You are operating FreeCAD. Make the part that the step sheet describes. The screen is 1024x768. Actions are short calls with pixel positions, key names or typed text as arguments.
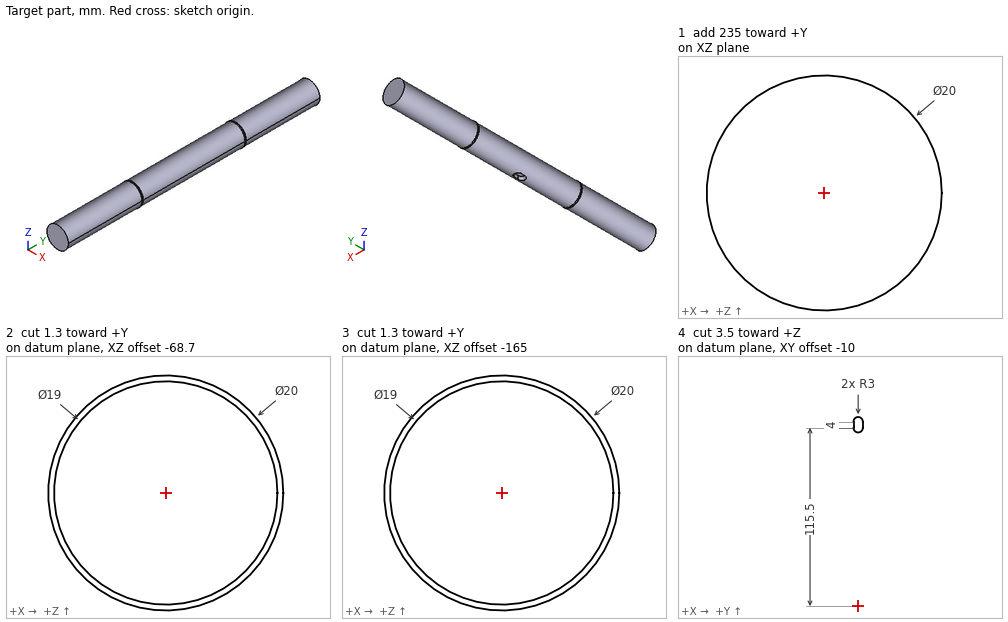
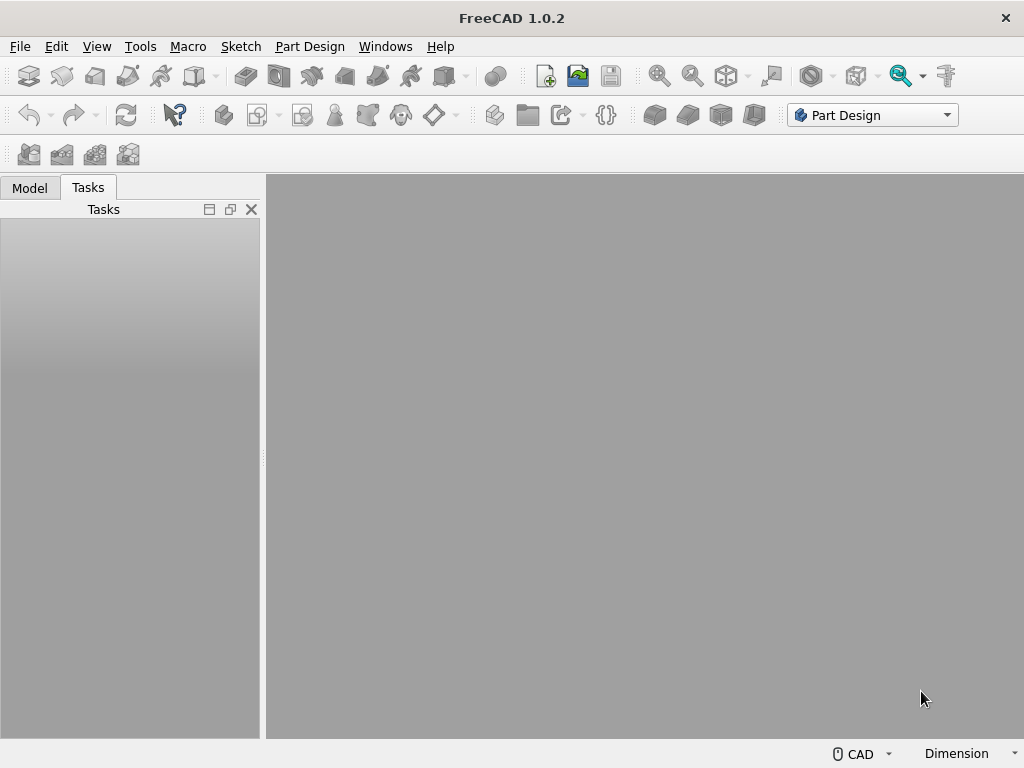
click(545, 76)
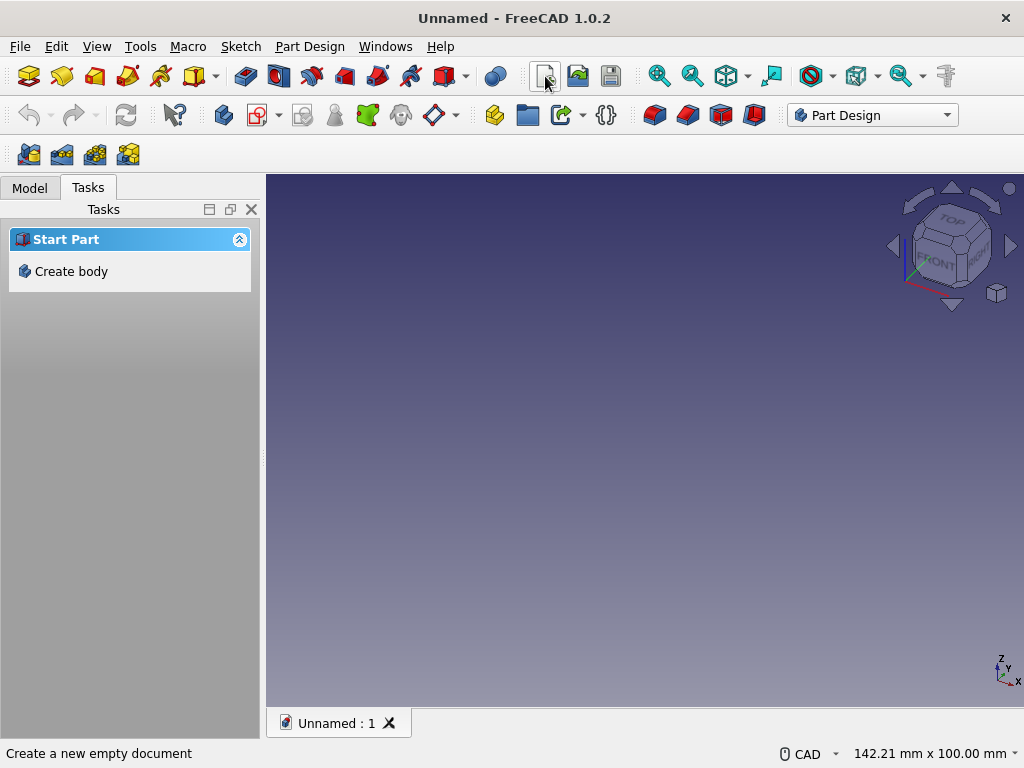
click(256, 116)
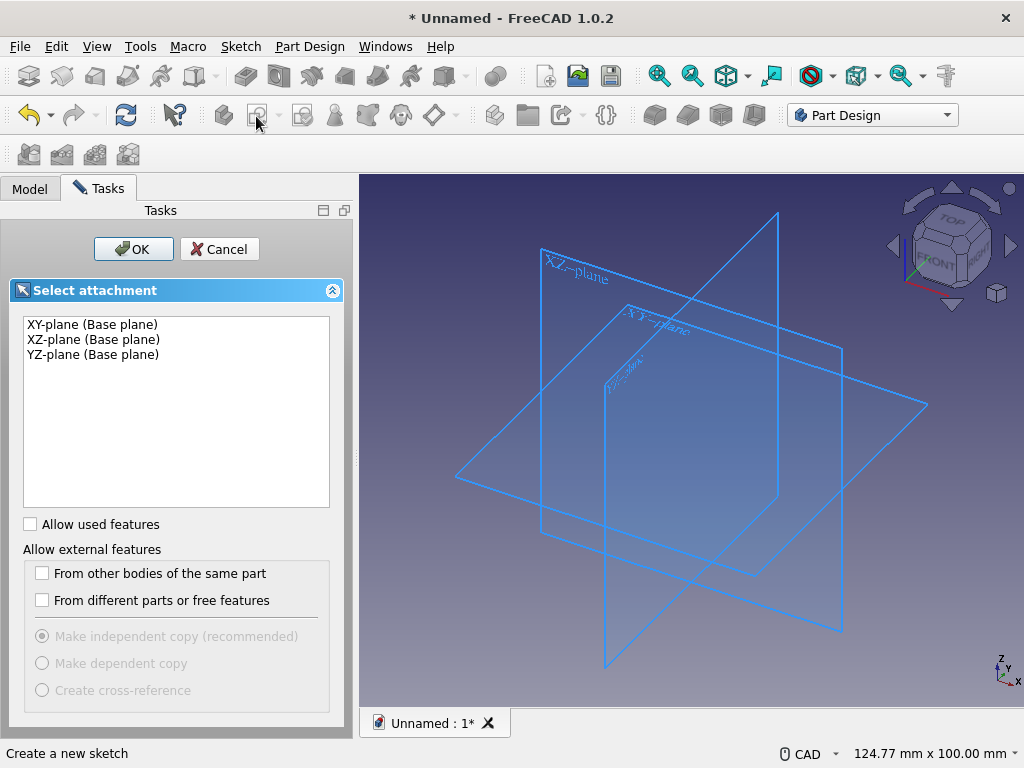
click(84, 340)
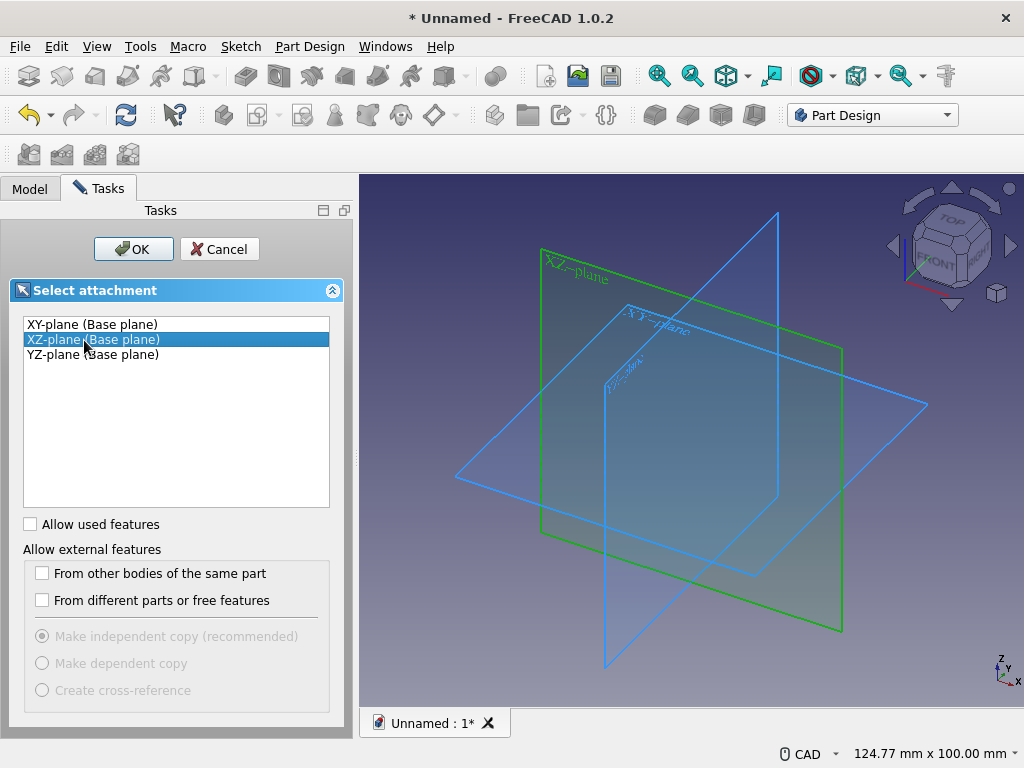
click(134, 249)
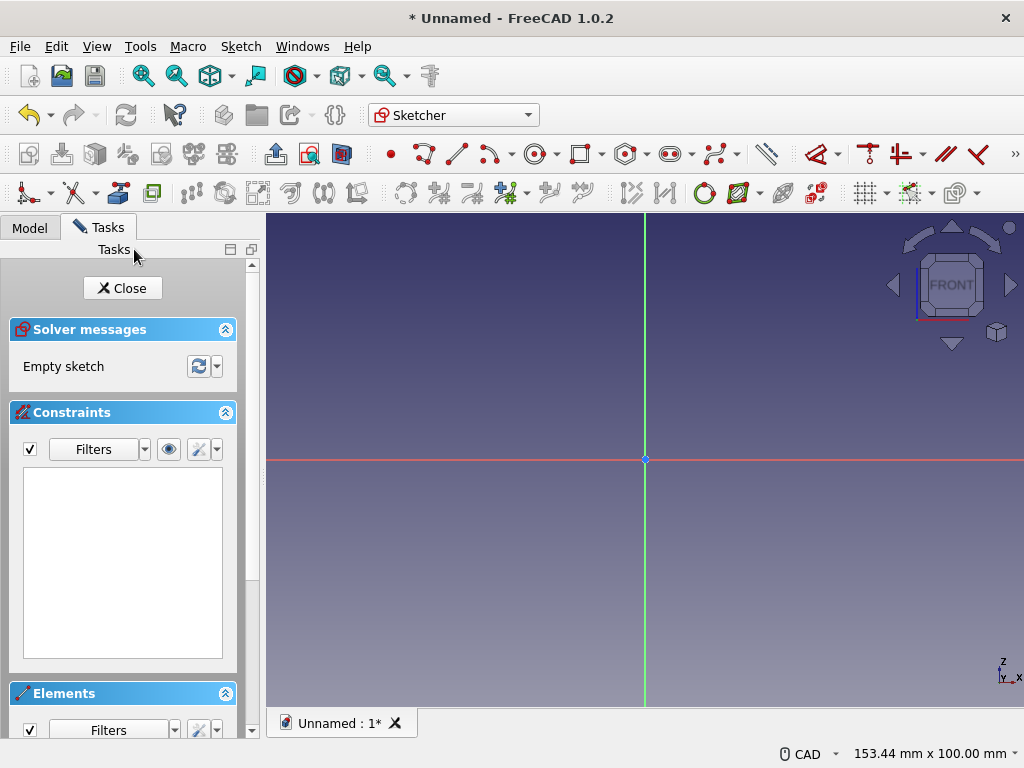
scroll(675, 460, up, 6)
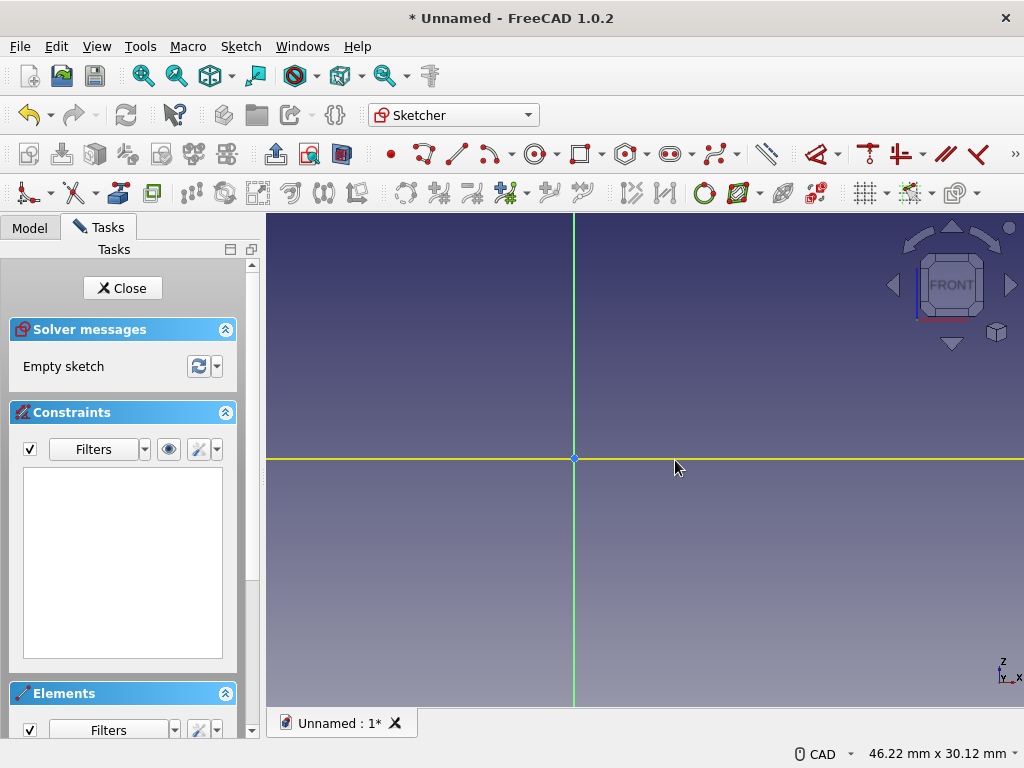
click(534, 154)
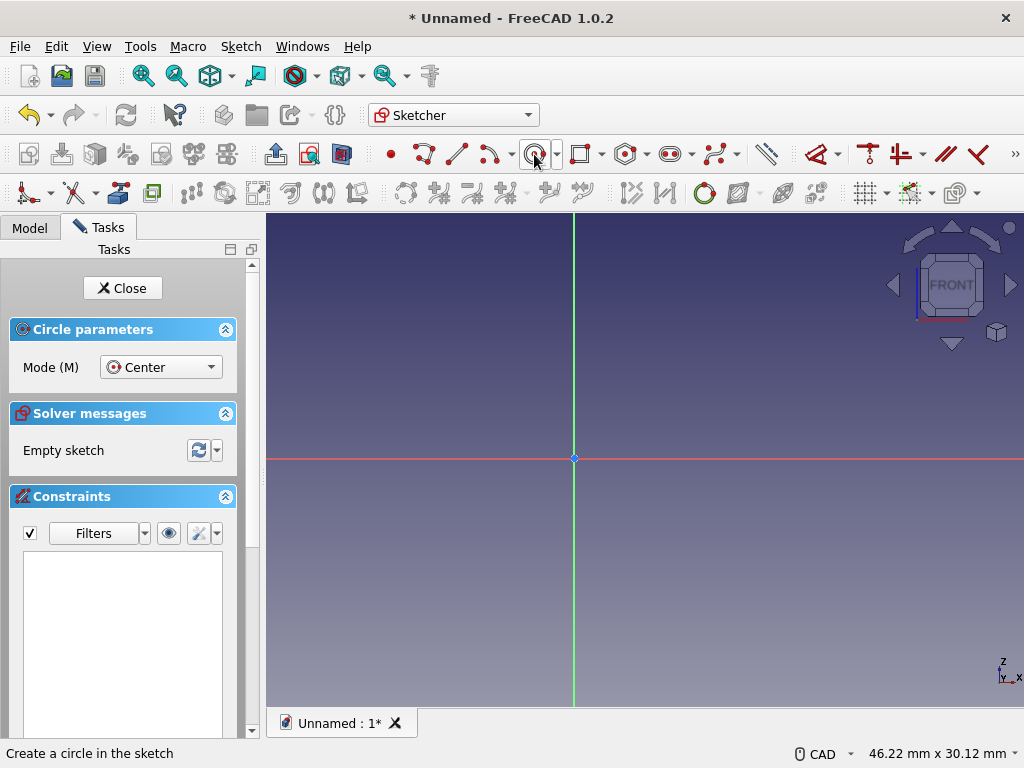
click(574, 459)
move(690, 343)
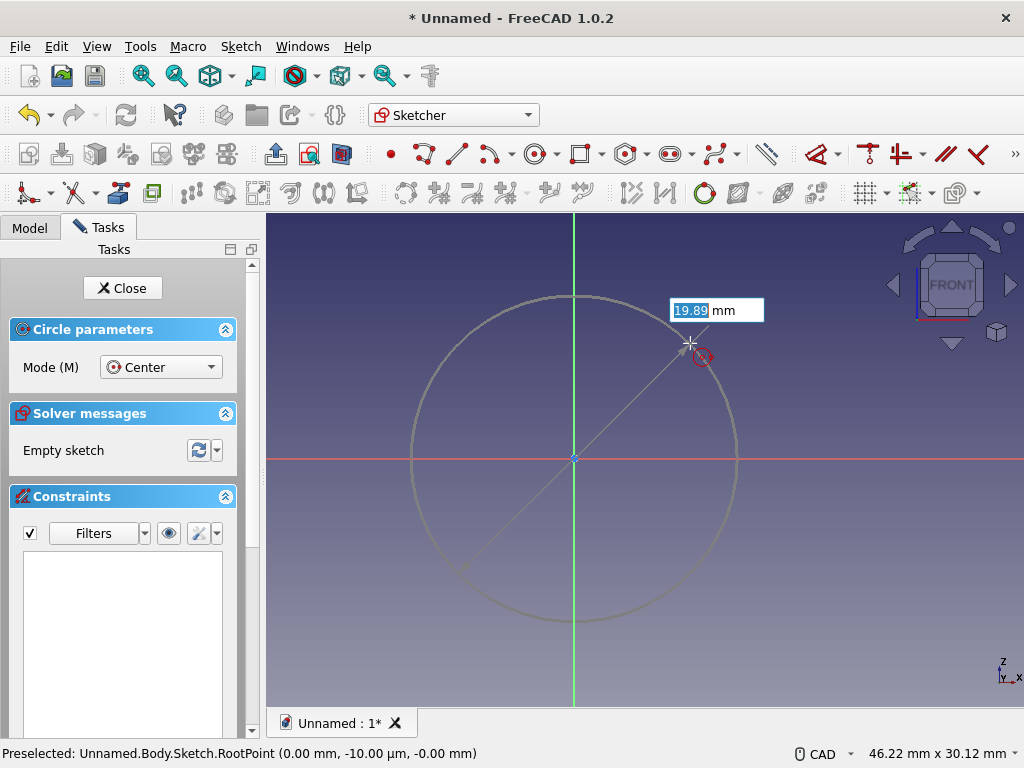
text(20)
key(Return)
key(Escape)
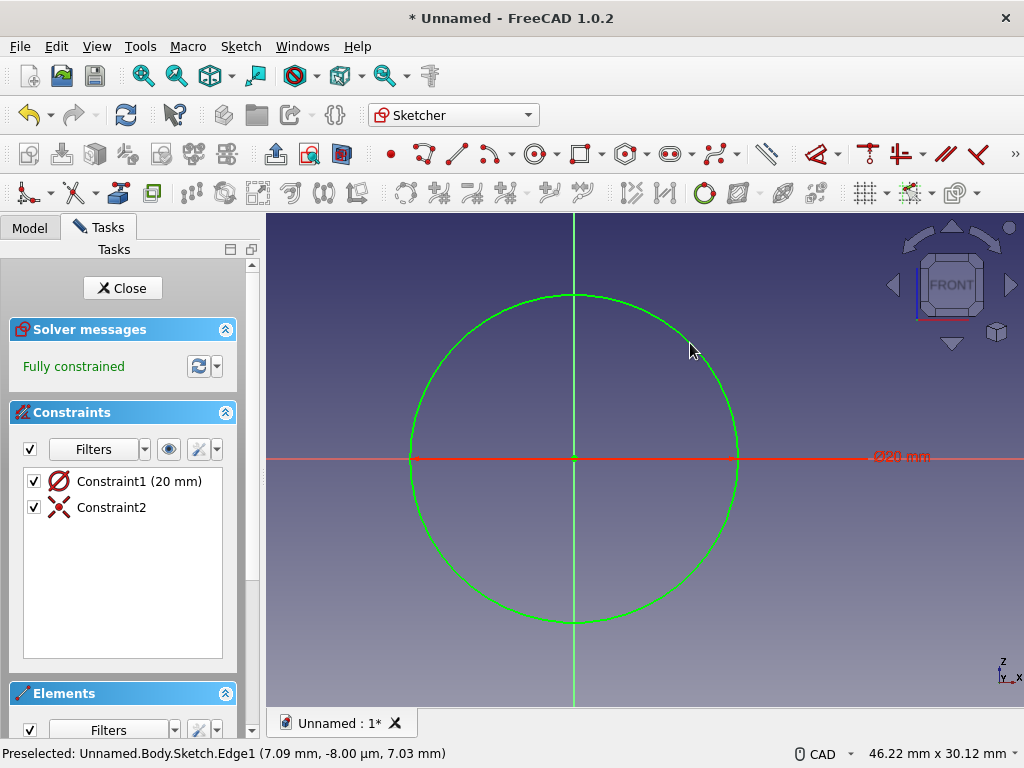
click(123, 288)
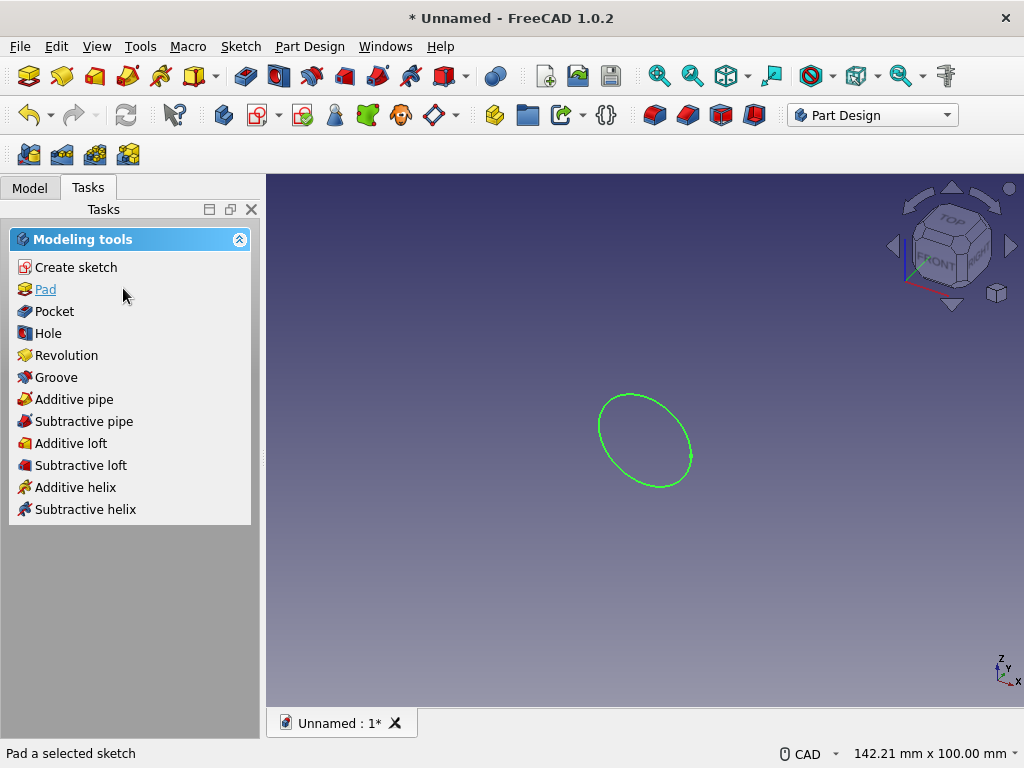
click(29, 76)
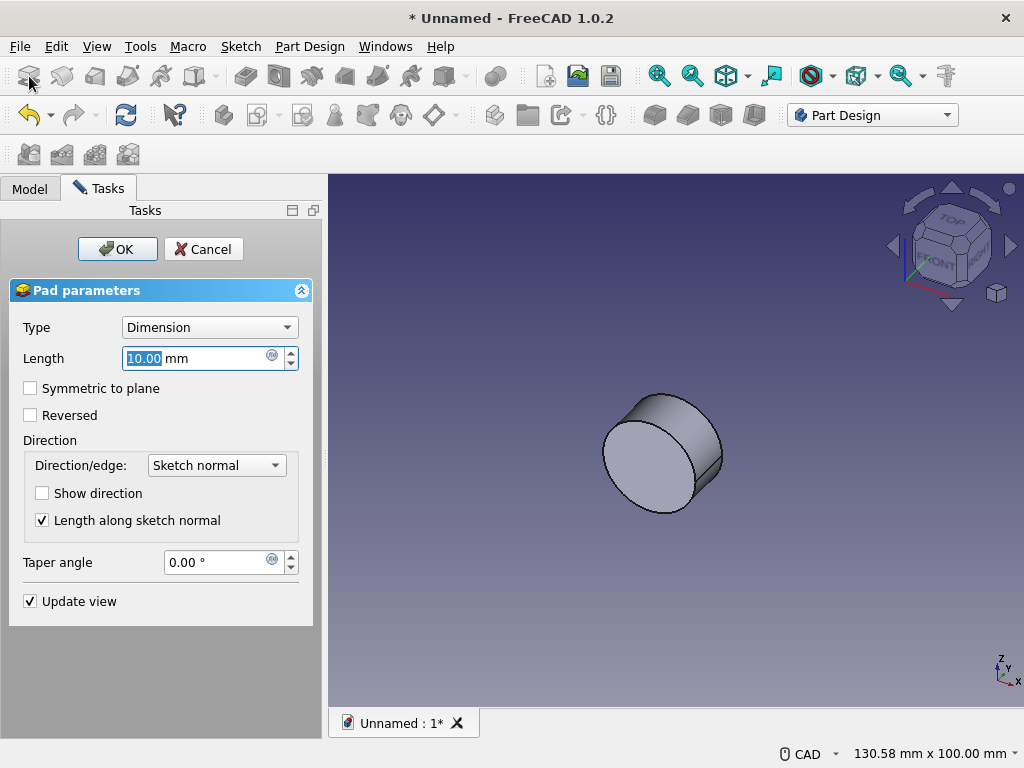
text(235)
key(Tab)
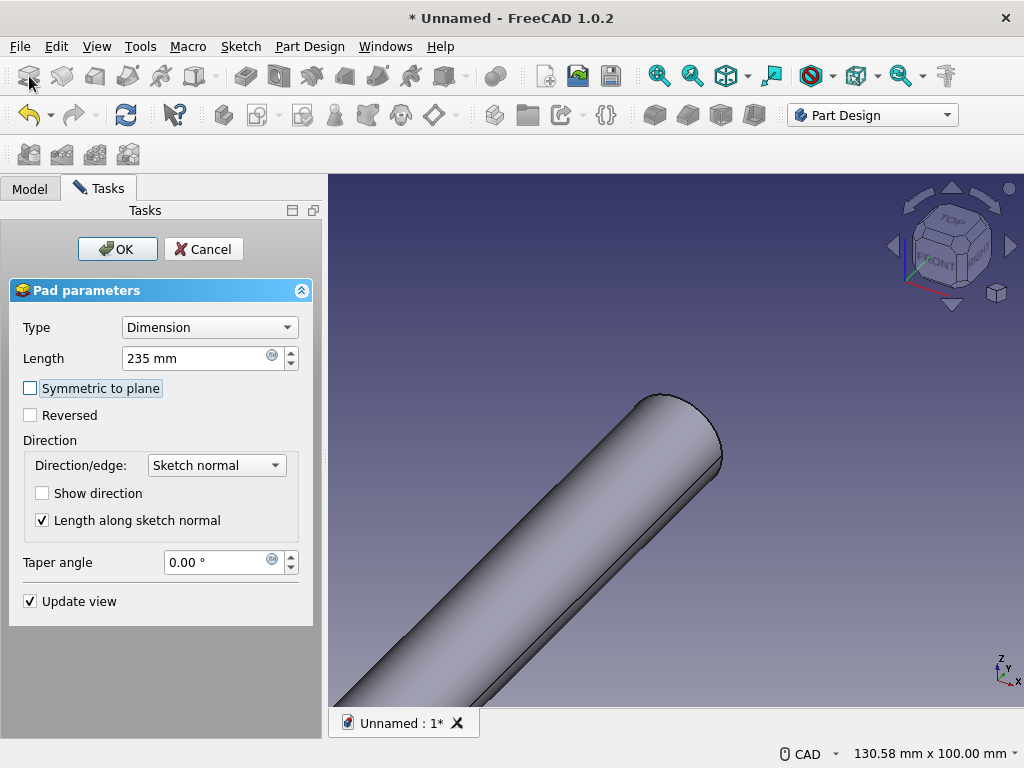
click(31, 415)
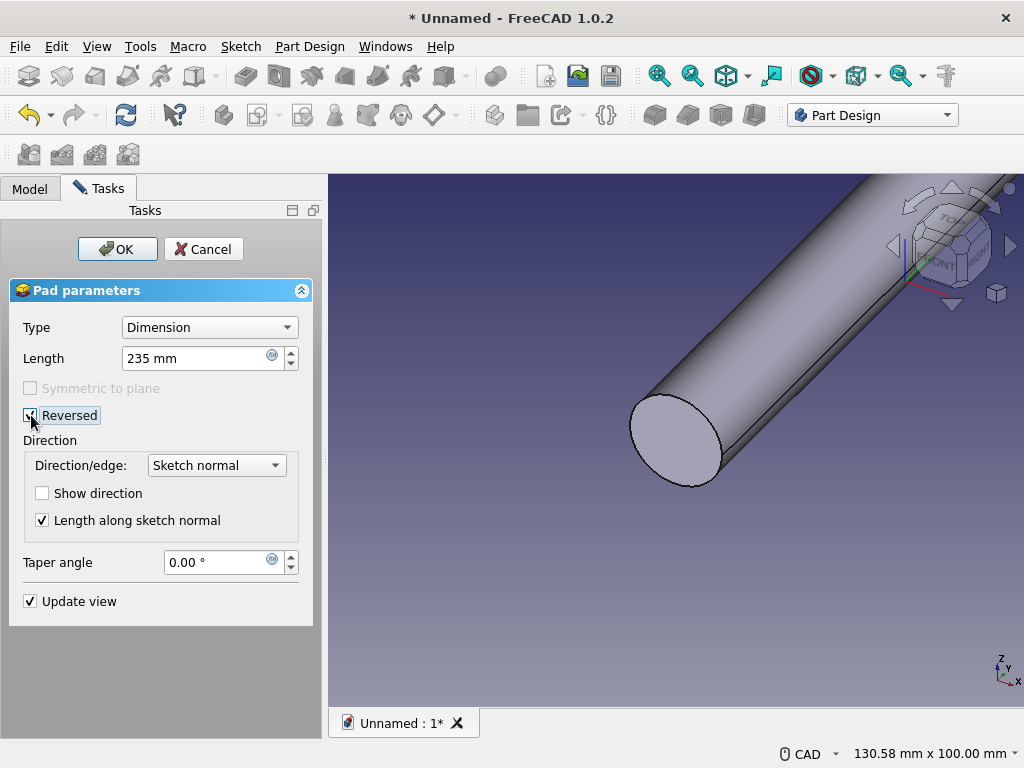
click(118, 249)